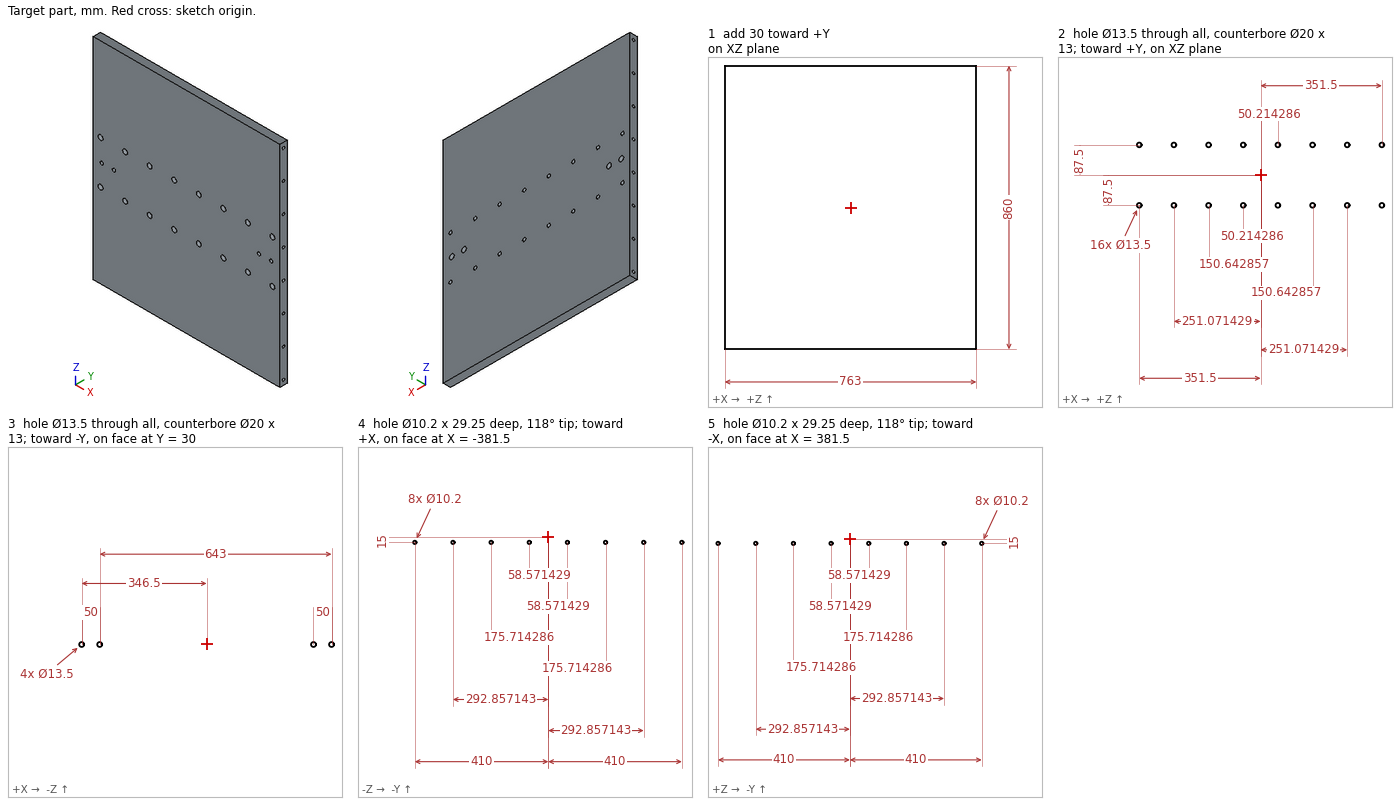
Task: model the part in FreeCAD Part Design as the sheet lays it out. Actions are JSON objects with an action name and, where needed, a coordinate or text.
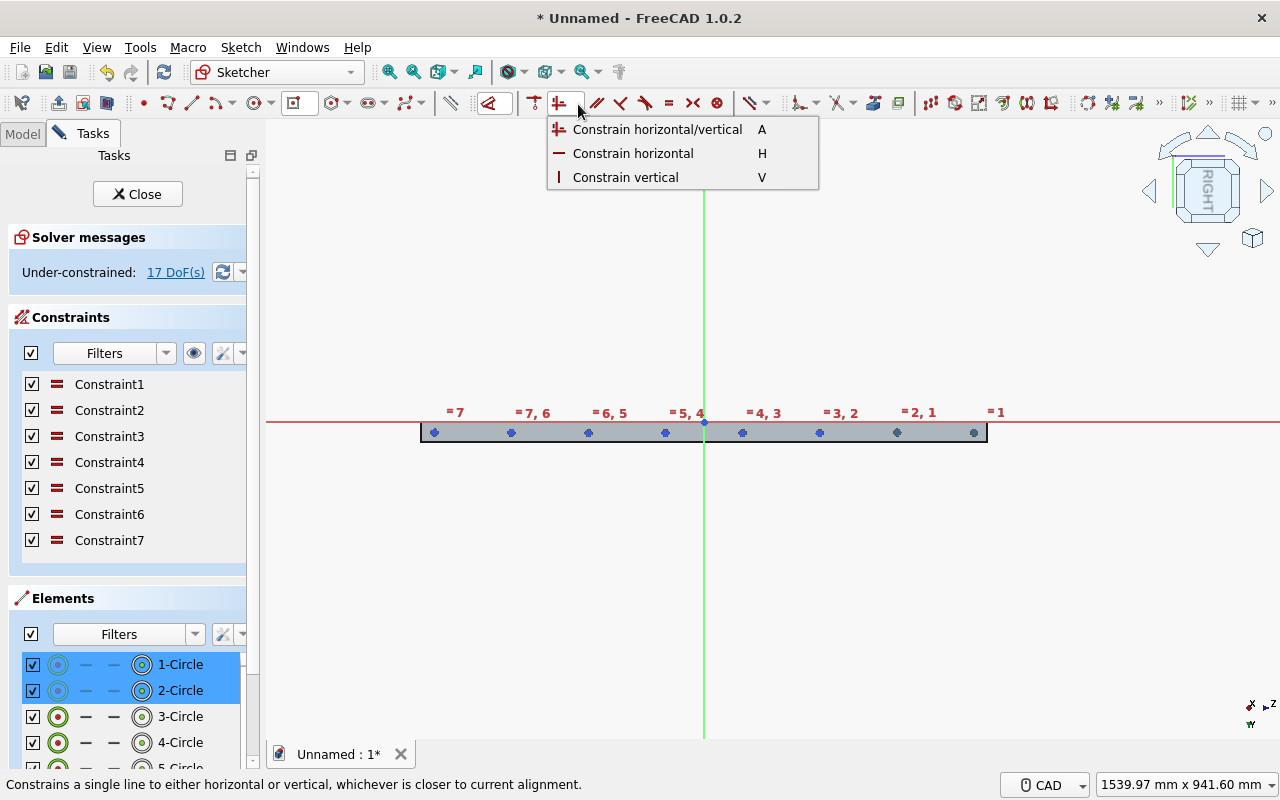
{"action": "left_click", "coordinate": [683, 153]}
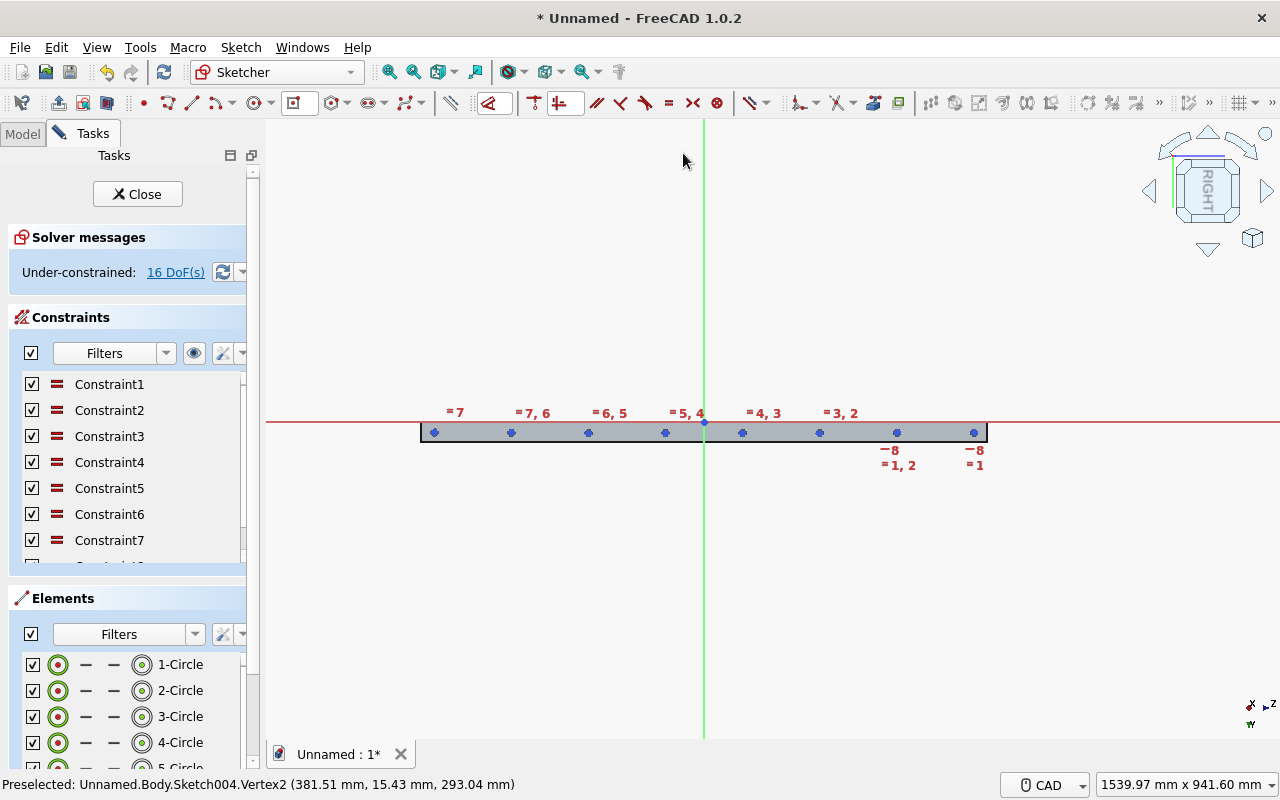
{"action": "left_click", "coordinate": [897, 433]}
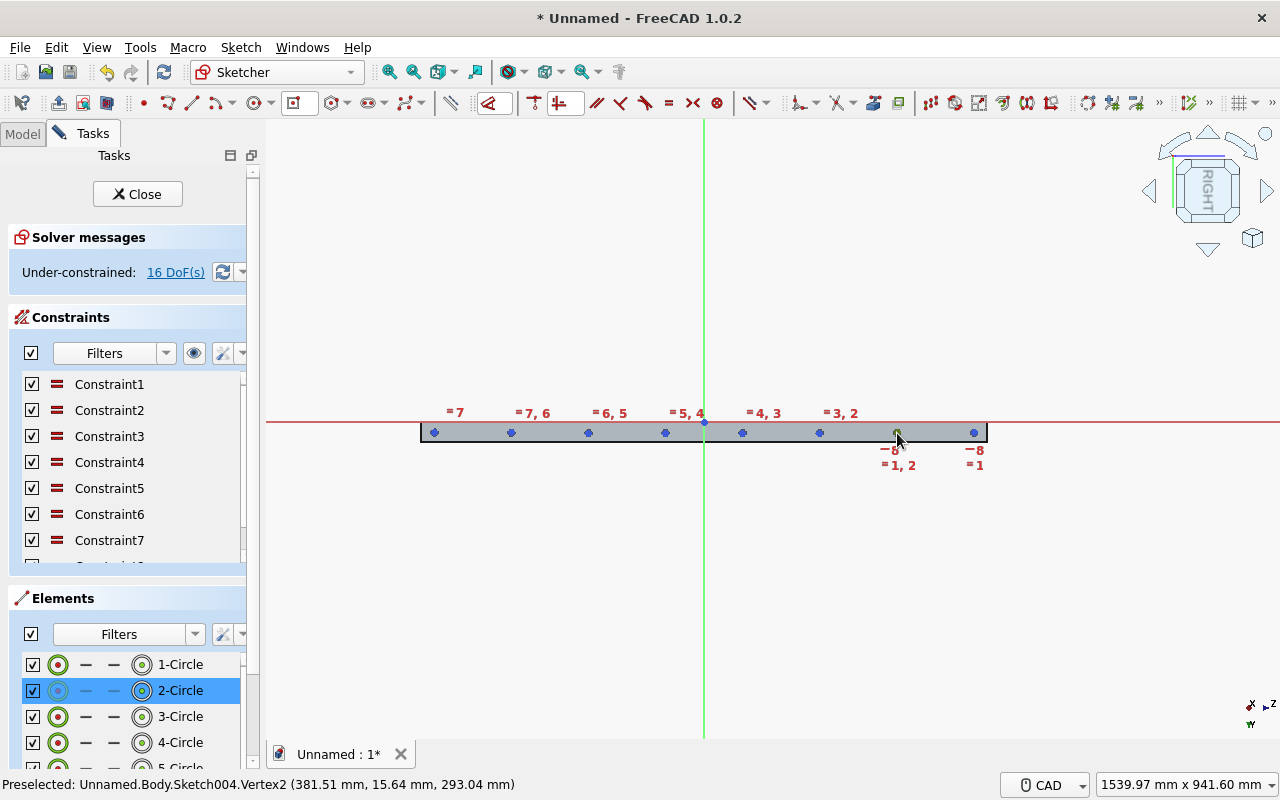
{"action": "left_click", "coordinate": [820, 433]}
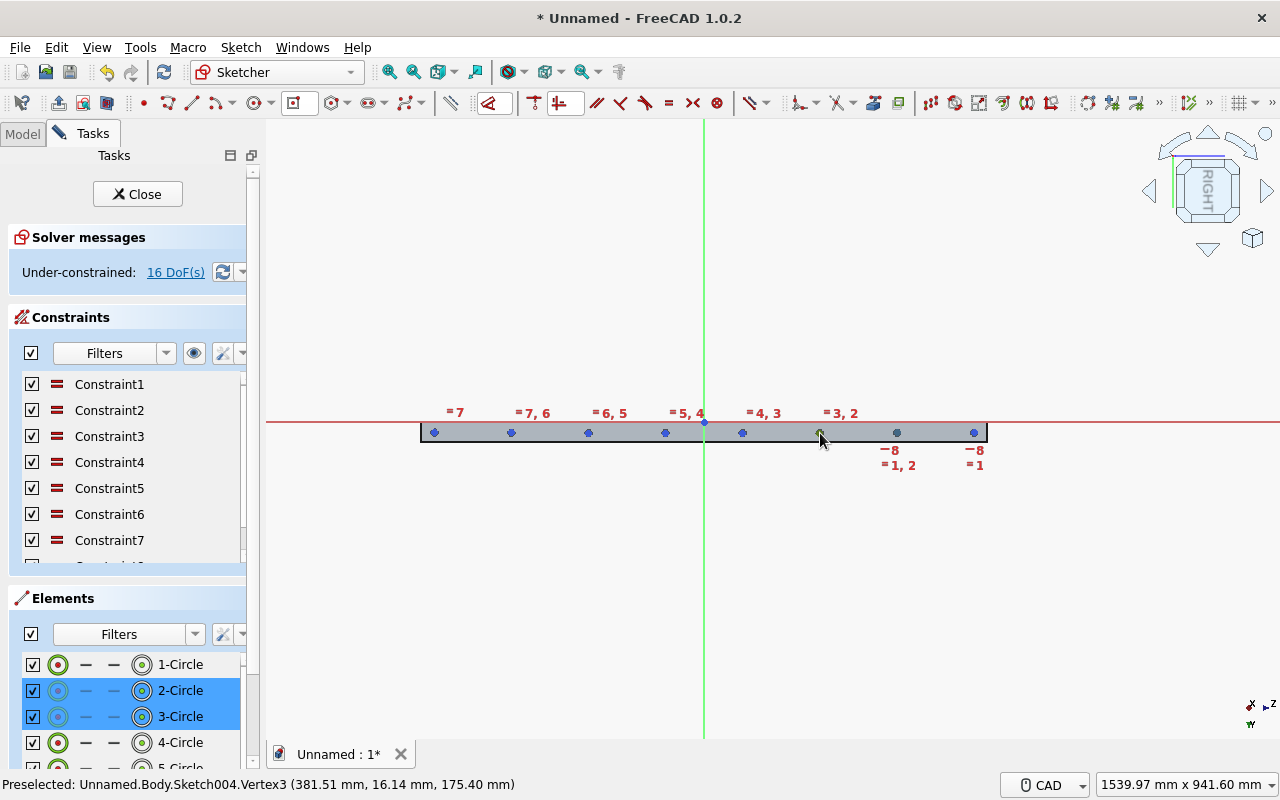
{"action": "left_click", "coordinate": [578, 104]}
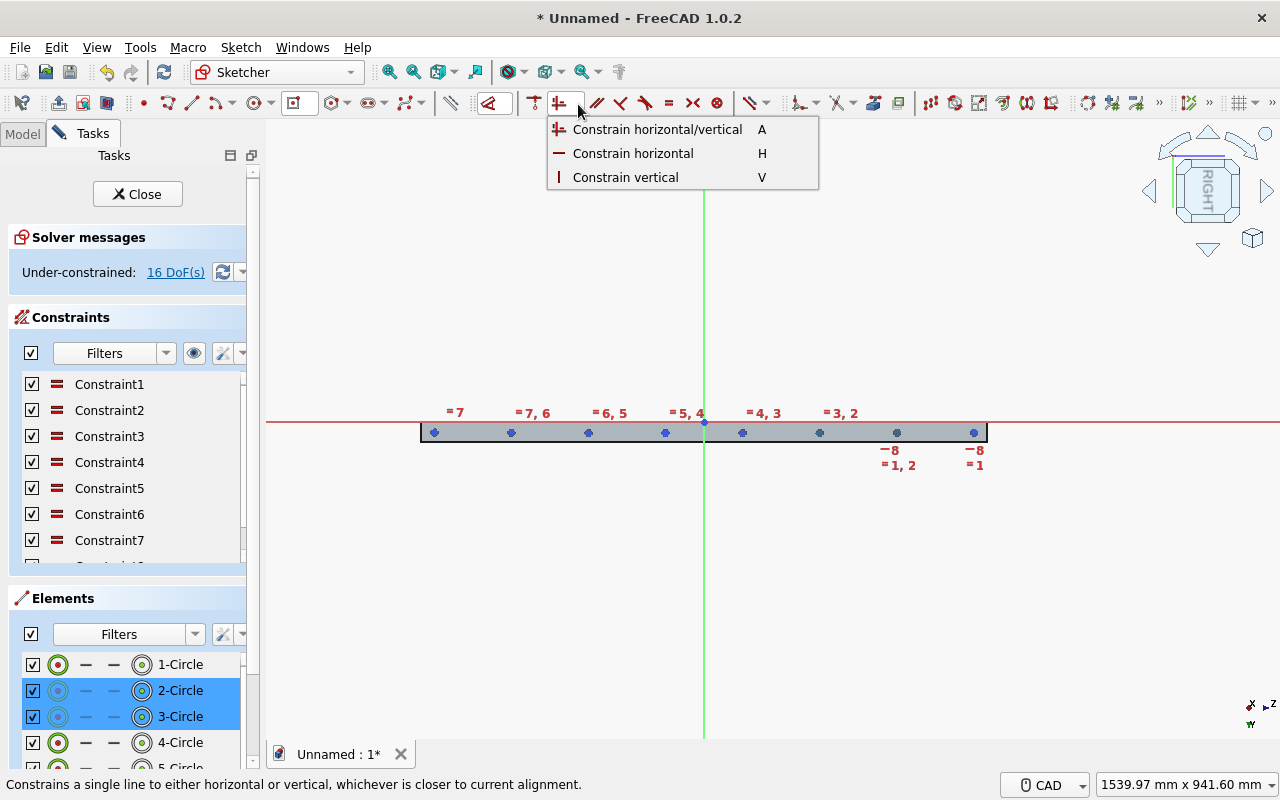
{"action": "left_click", "coordinate": [683, 153]}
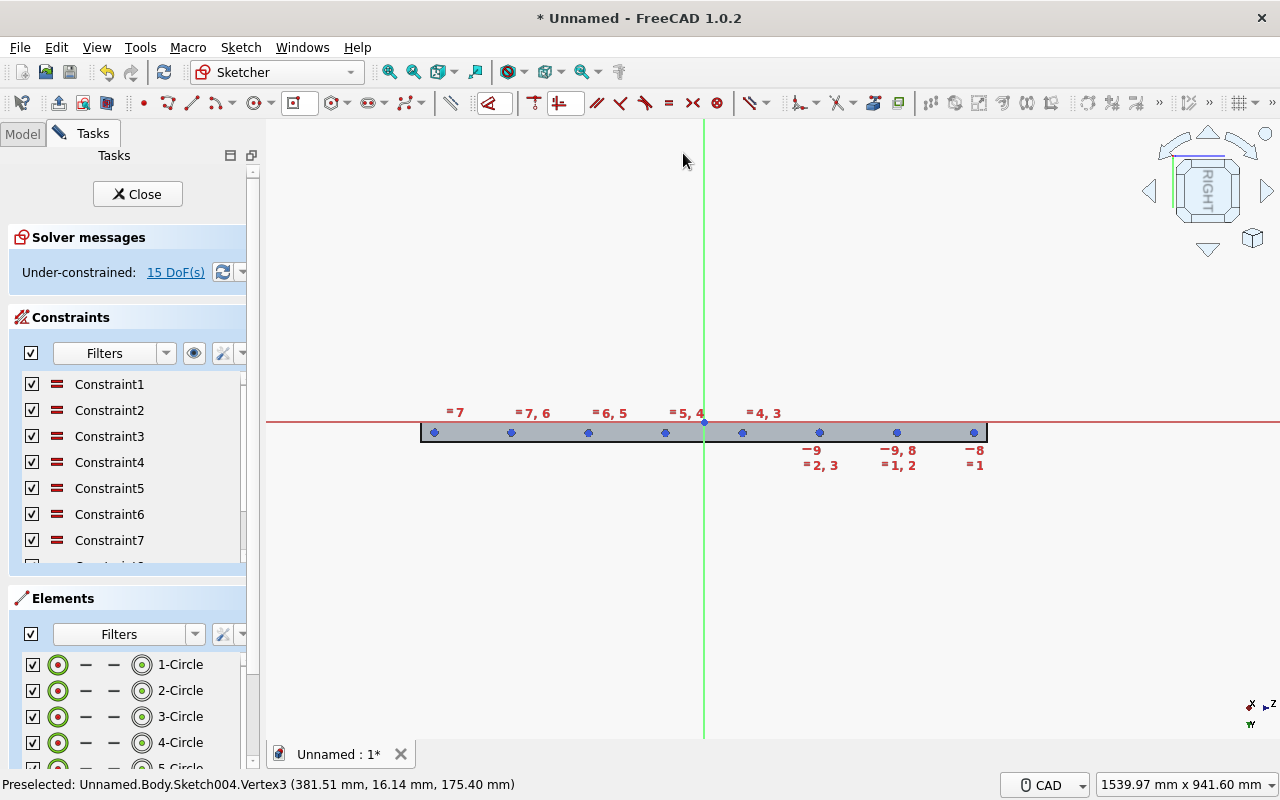
{"action": "left_click", "coordinate": [820, 433]}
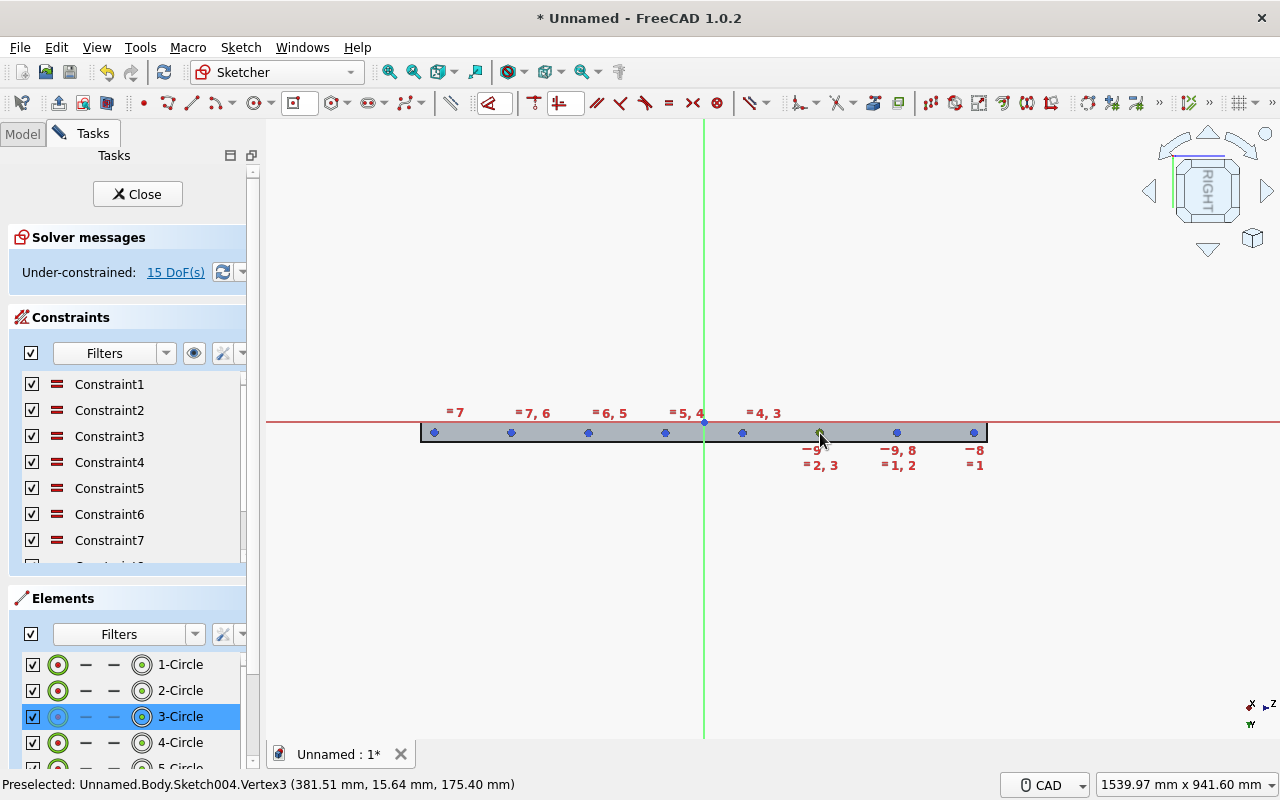
{"action": "left_click", "coordinate": [743, 433]}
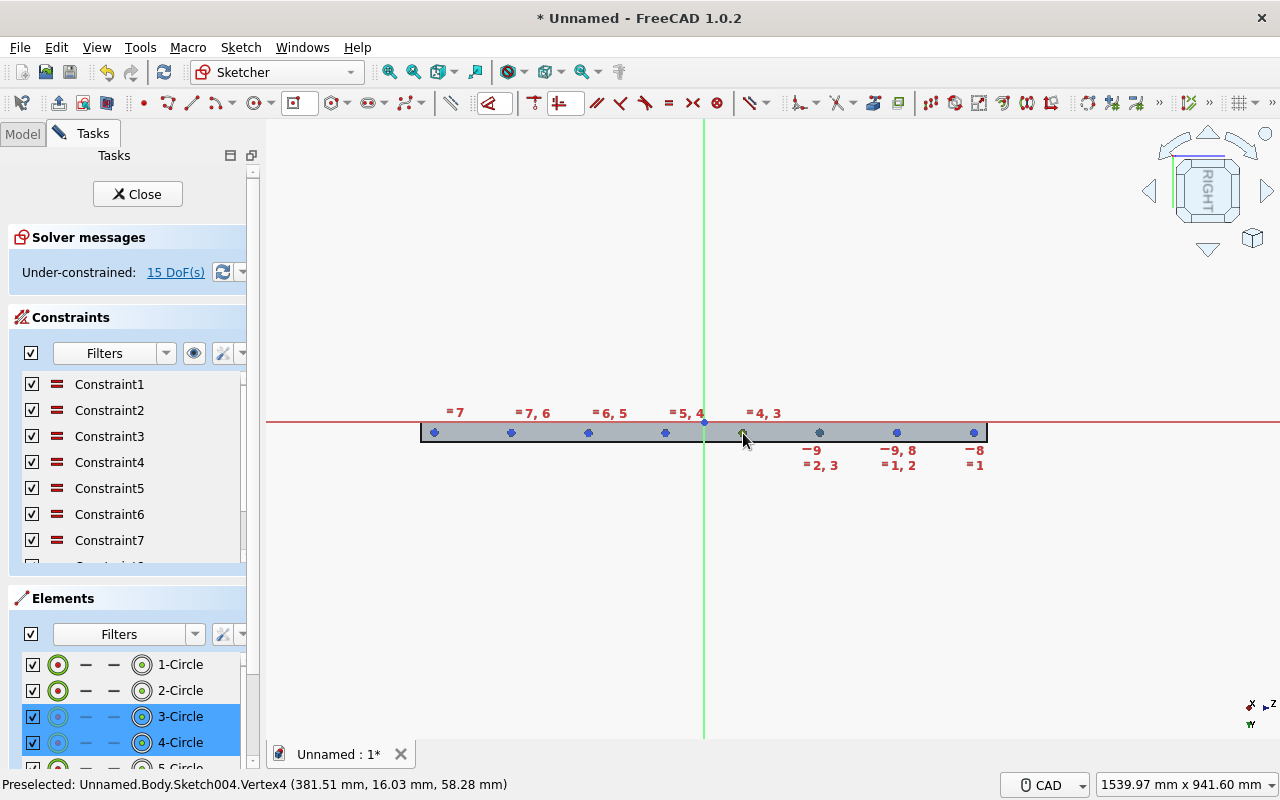
{"action": "left_click", "coordinate": [578, 104]}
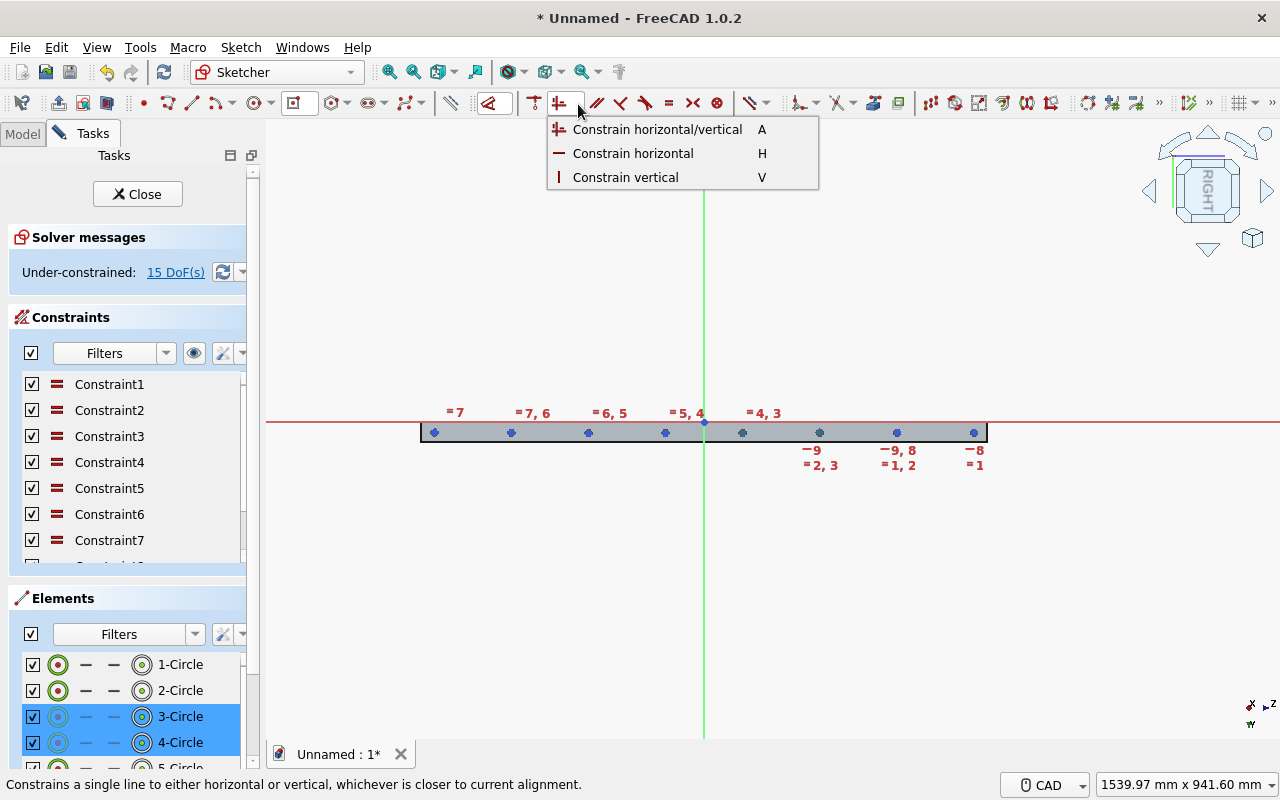
{"action": "left_click", "coordinate": [683, 153]}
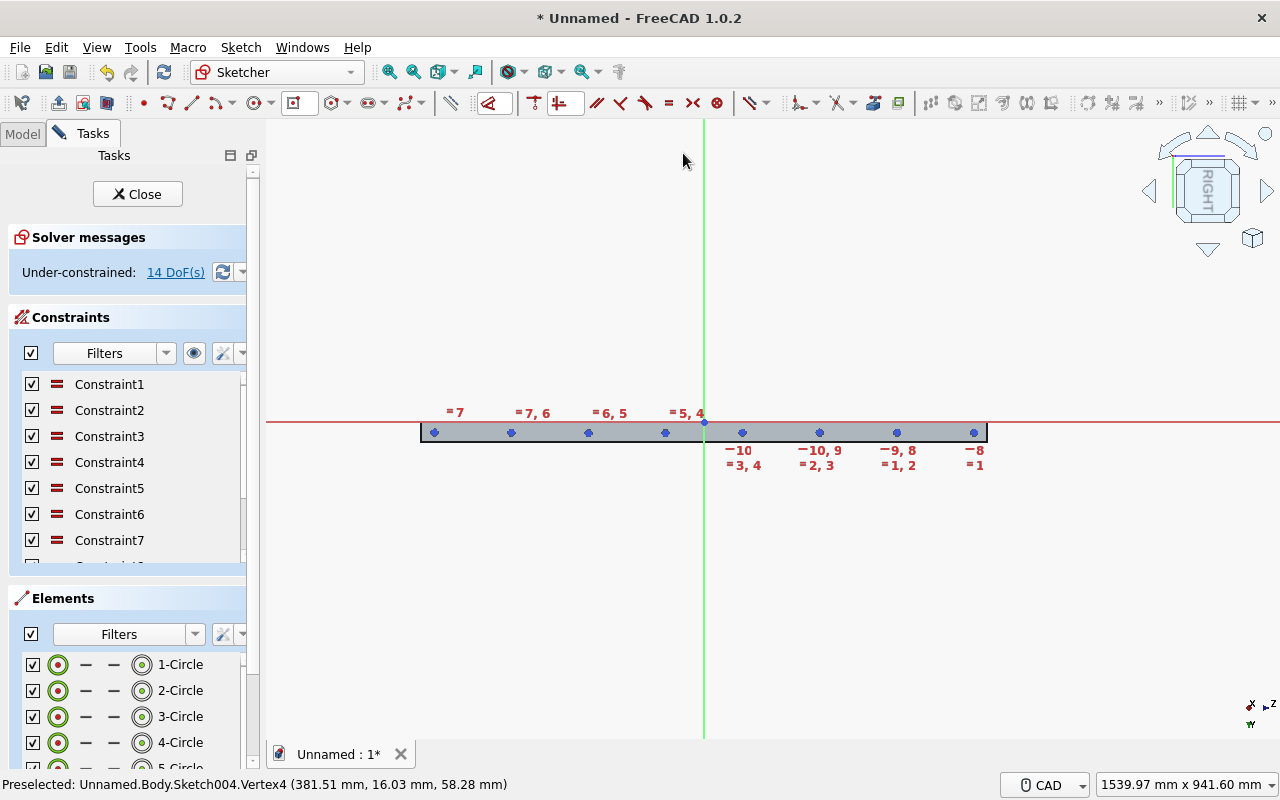
{"action": "left_click", "coordinate": [743, 433]}